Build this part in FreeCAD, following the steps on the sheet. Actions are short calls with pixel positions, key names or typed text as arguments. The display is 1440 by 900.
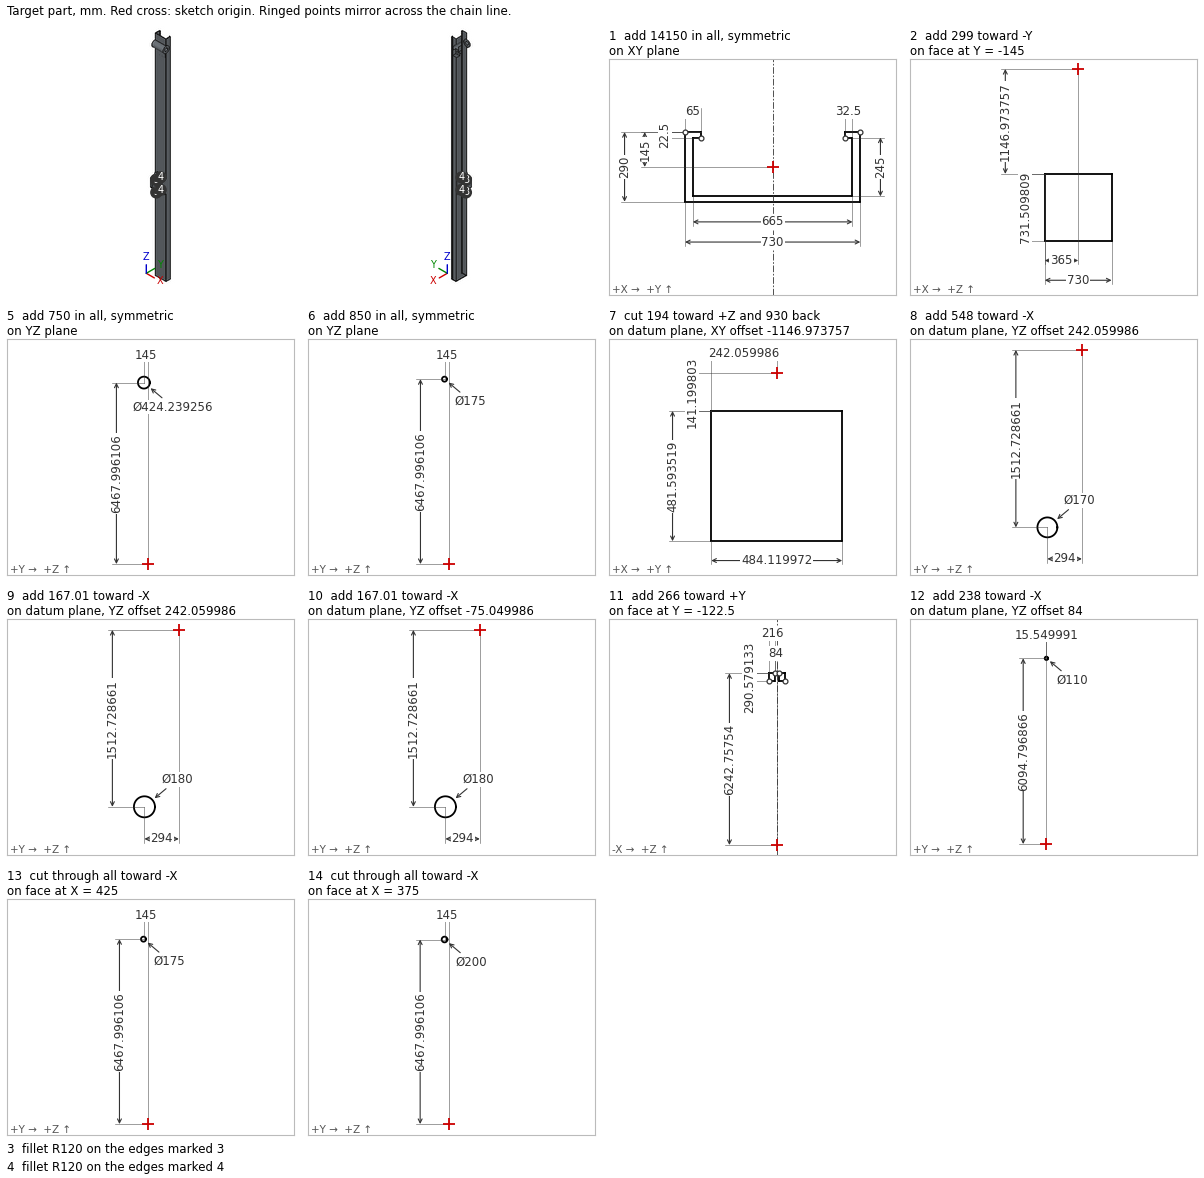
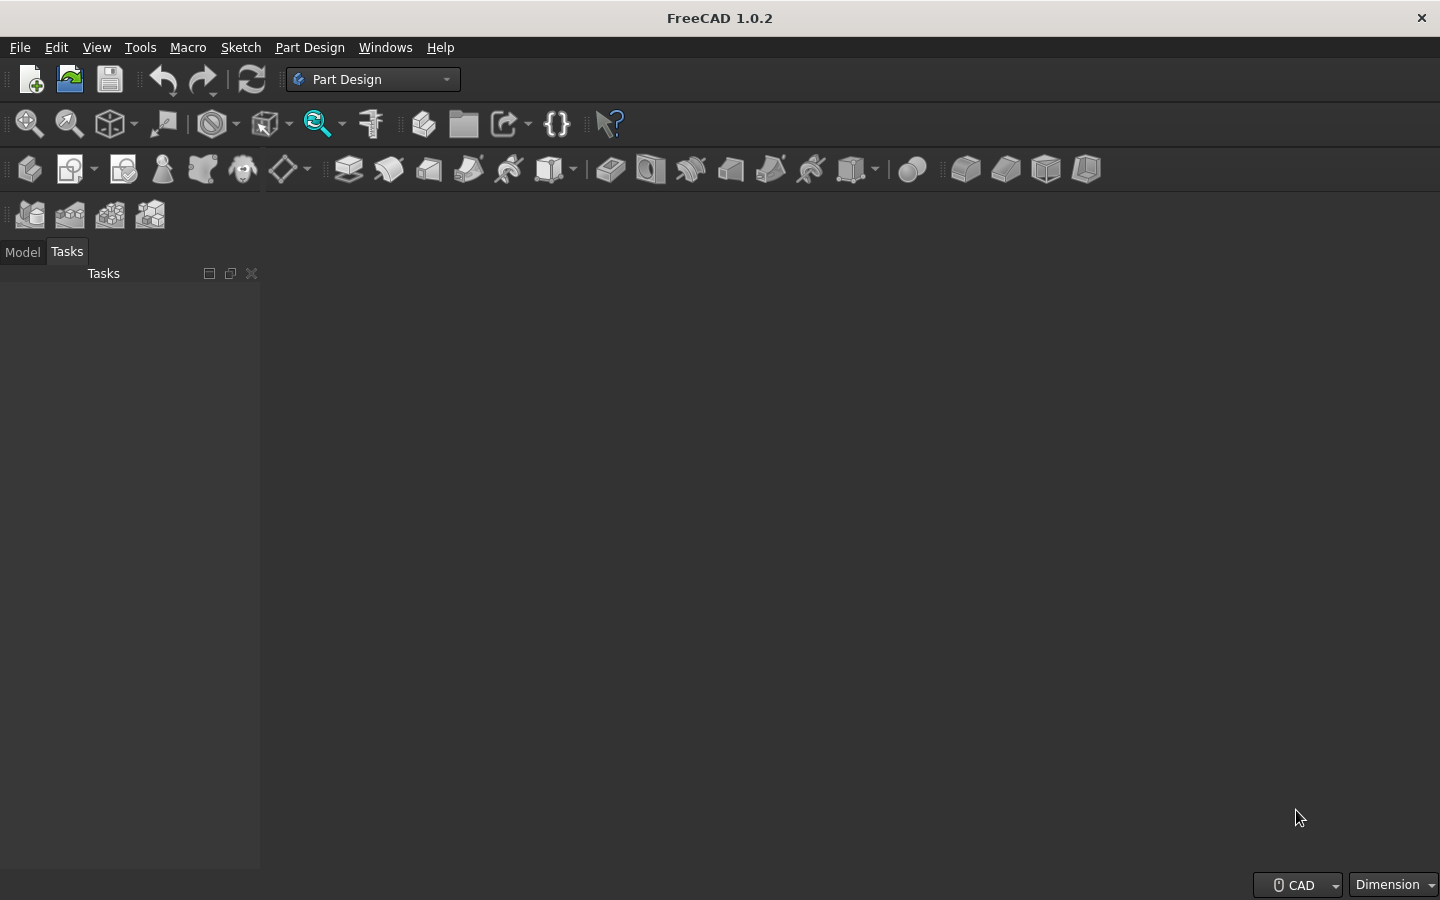
key(ctrl+n)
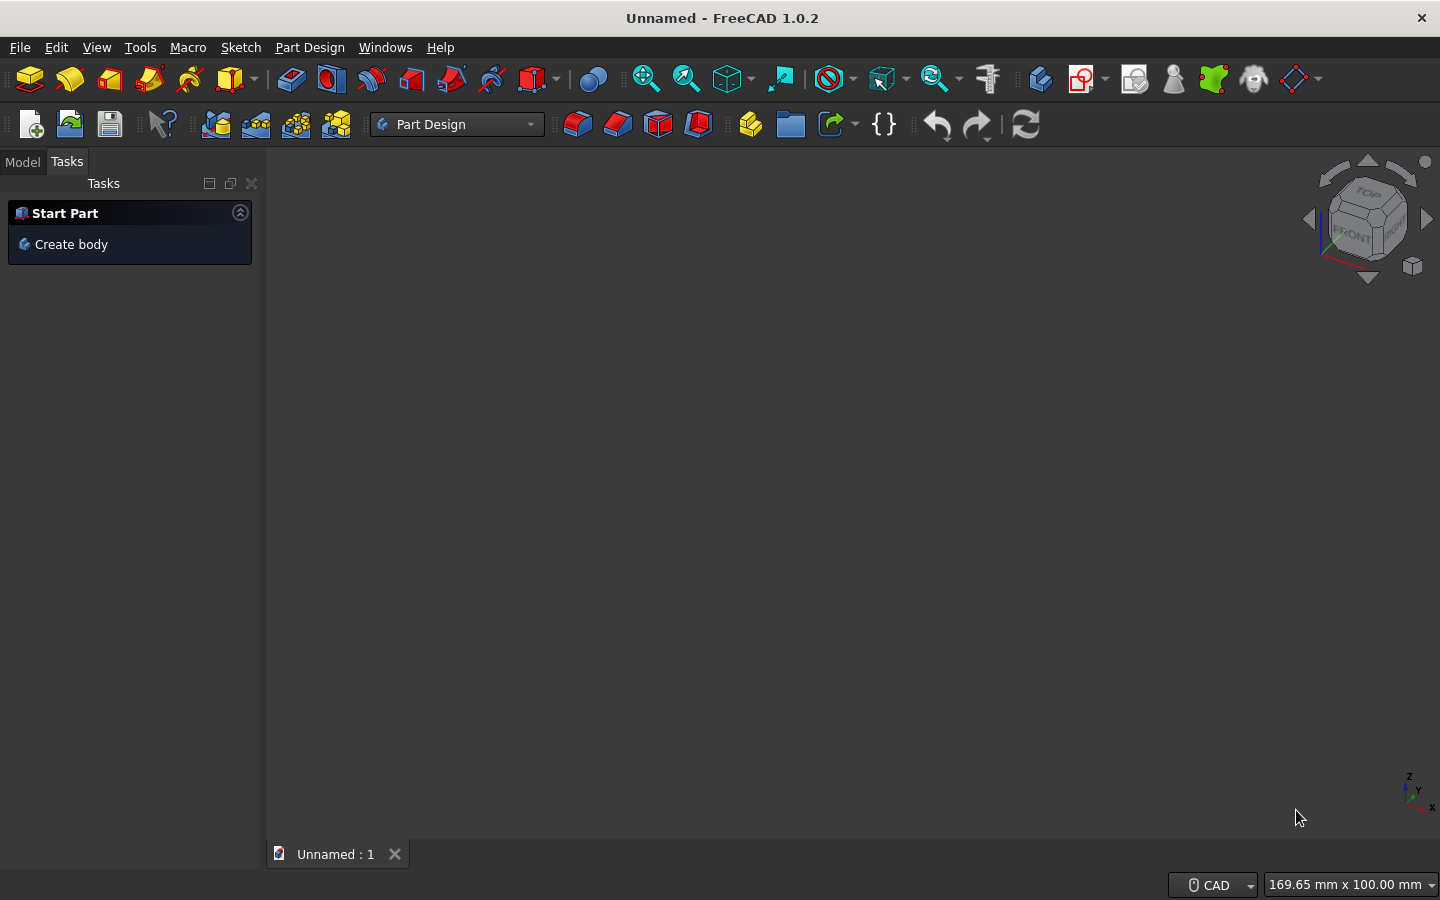
click(1082, 80)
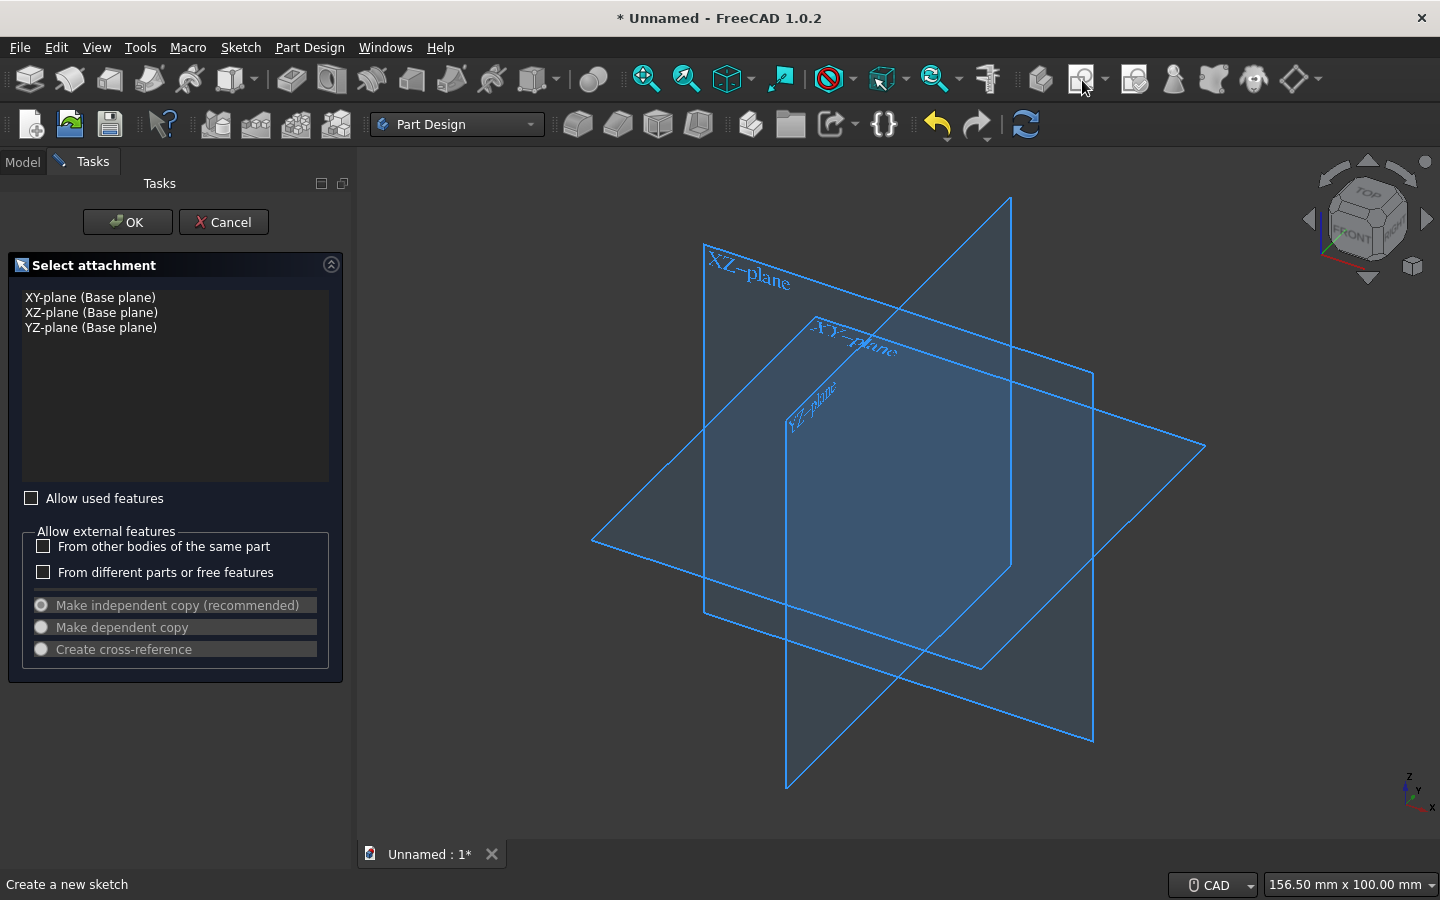
click(82, 298)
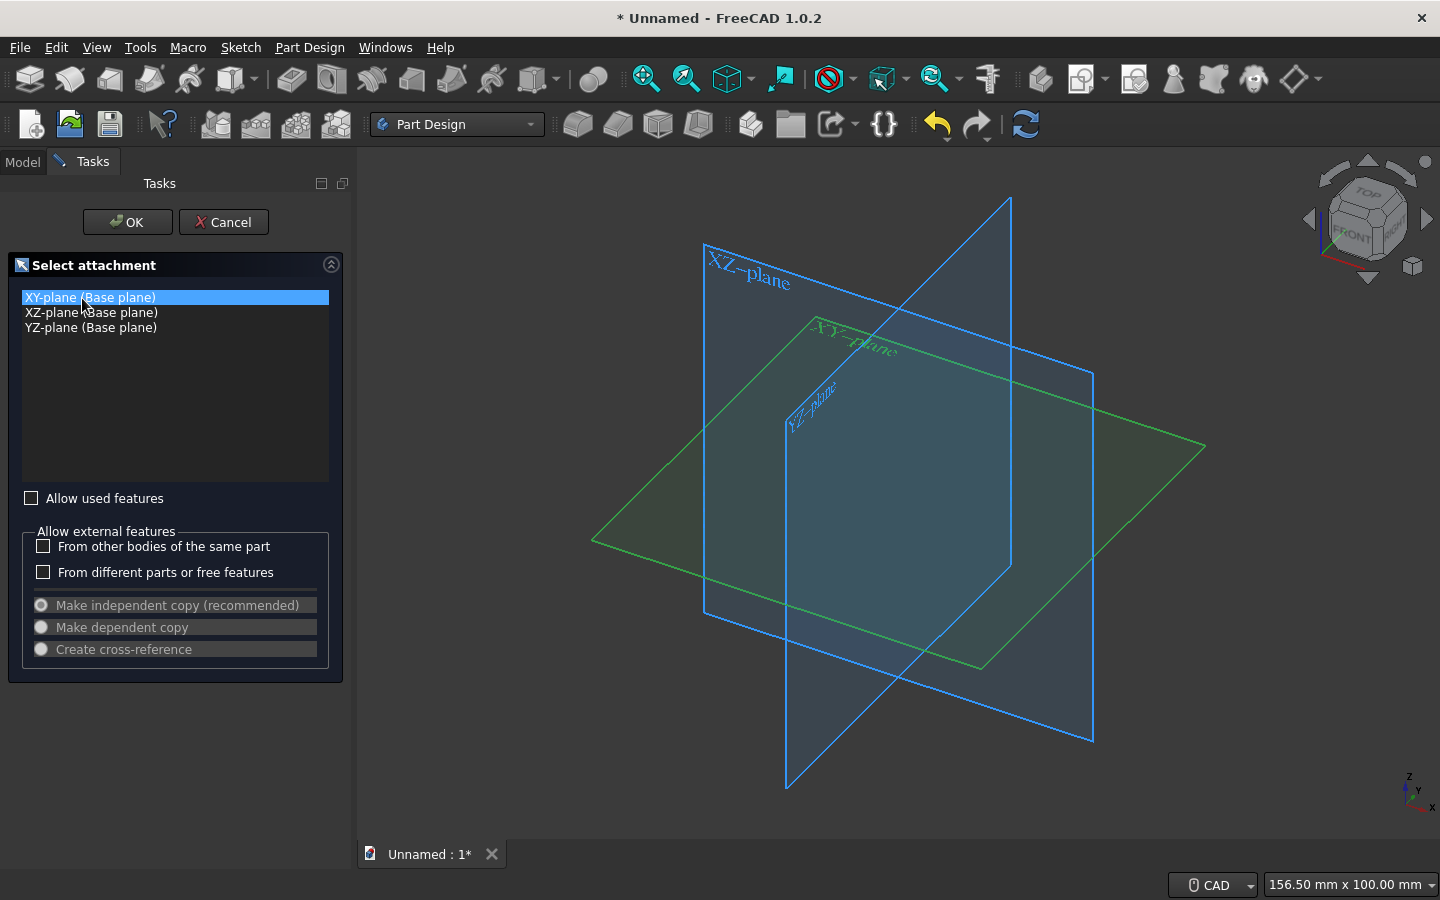
click(128, 222)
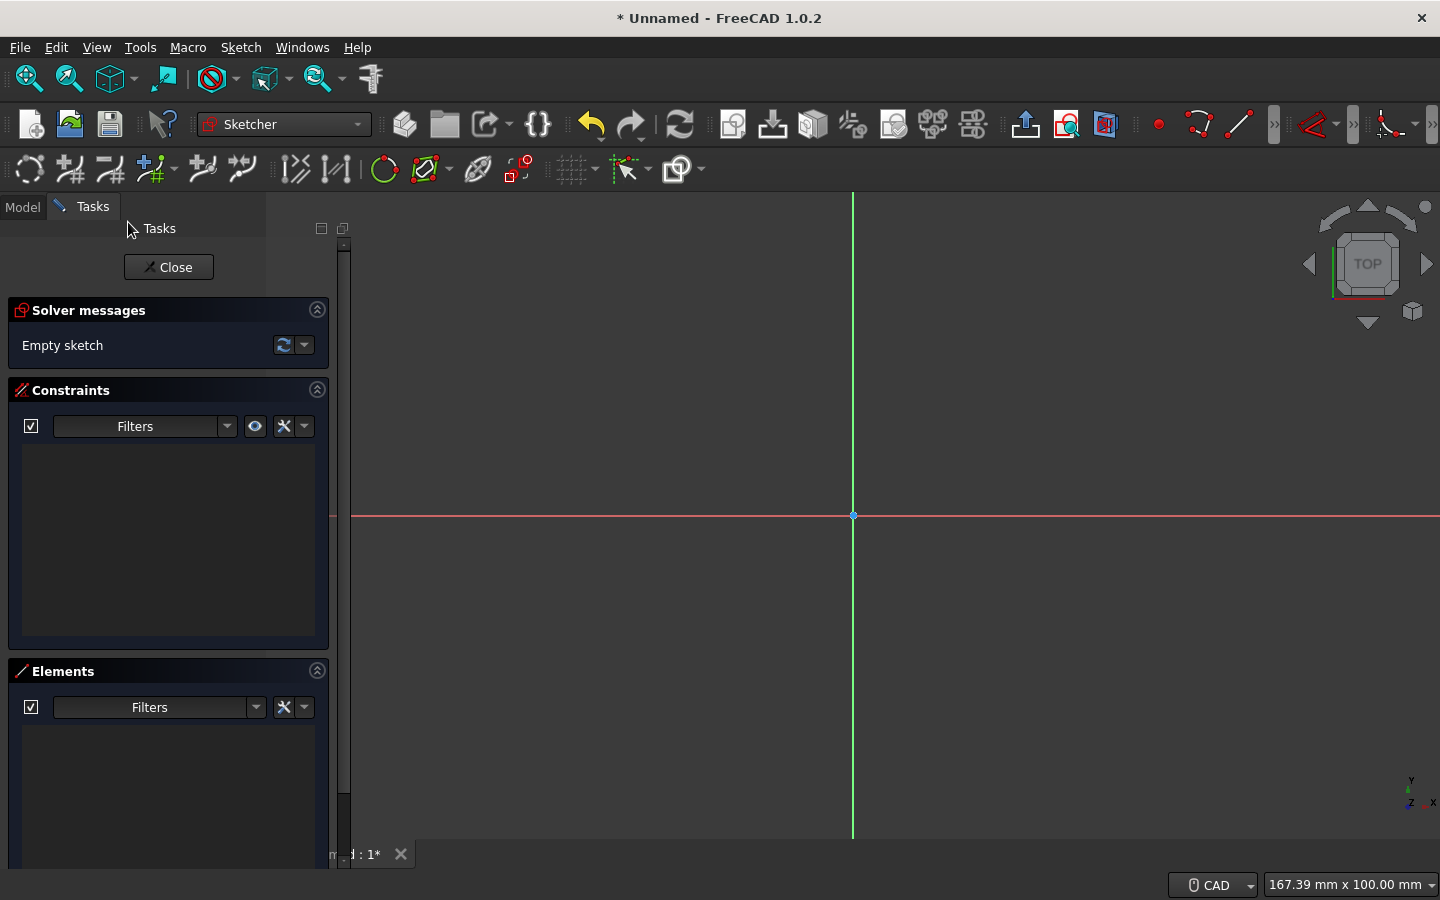
scroll(774, 516, down, 10)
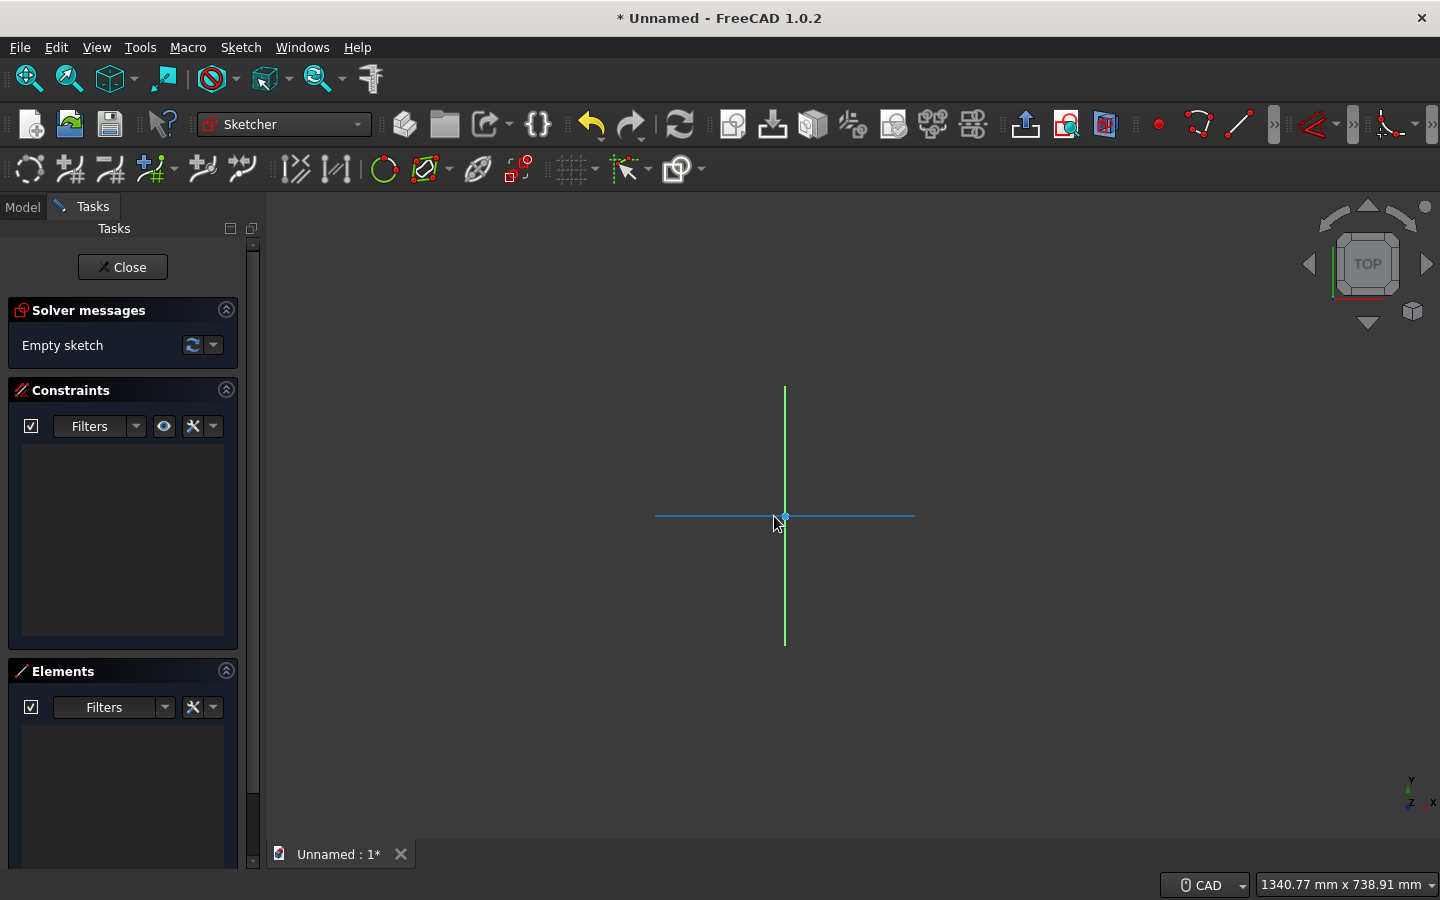
key(g)
key(m)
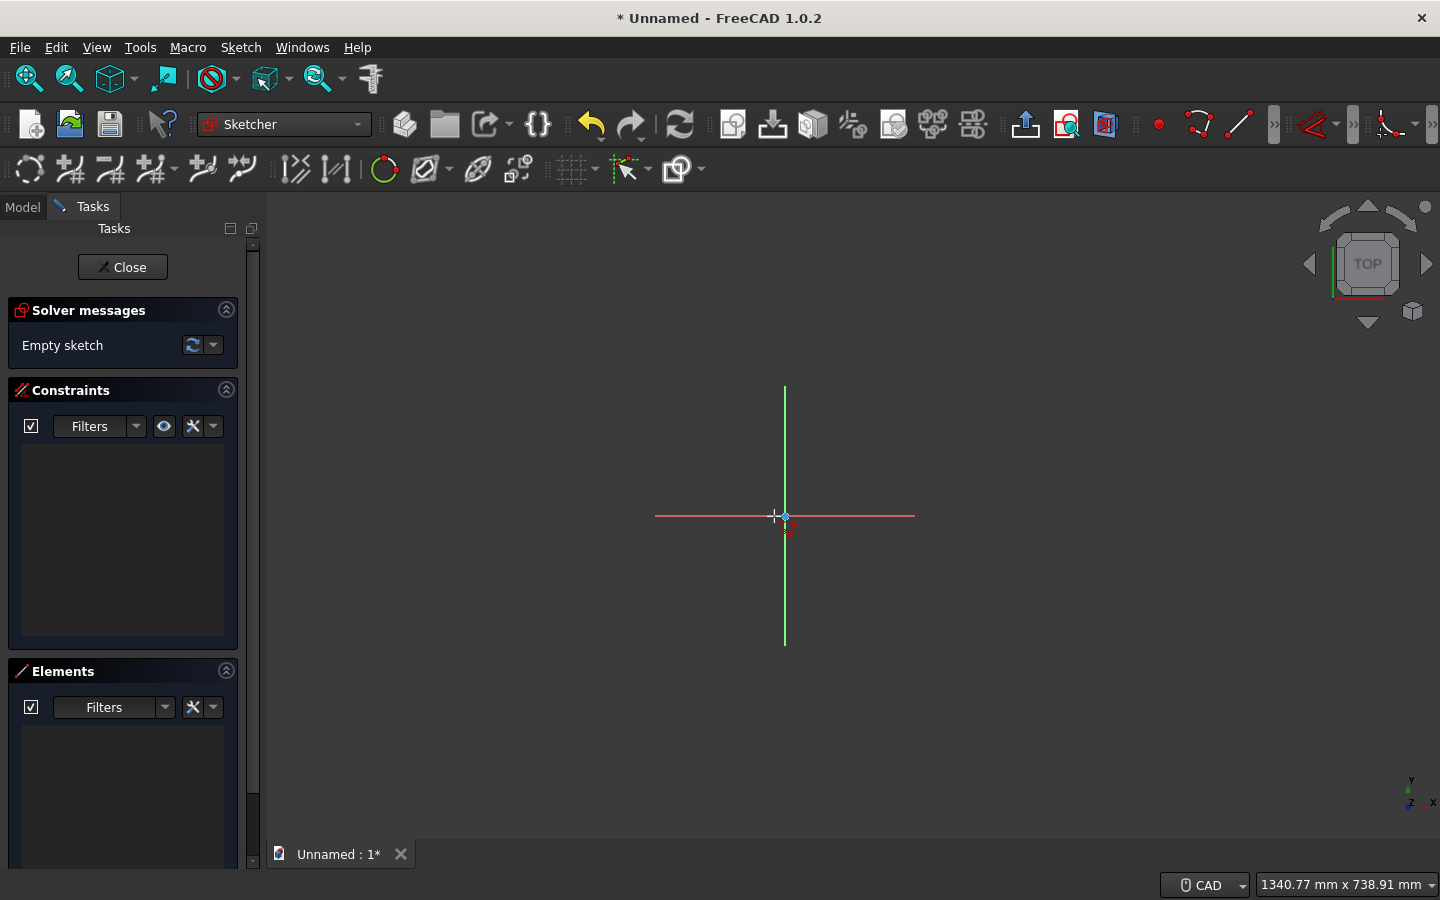
click(522, 409)
click(522, 389)
click(465, 389)
click(465, 643)
click(1105, 643)
click(1105, 389)
click(1048, 389)
click(1048, 409)
click(1076, 409)
click(1076, 624)
click(494, 624)
click(494, 409)